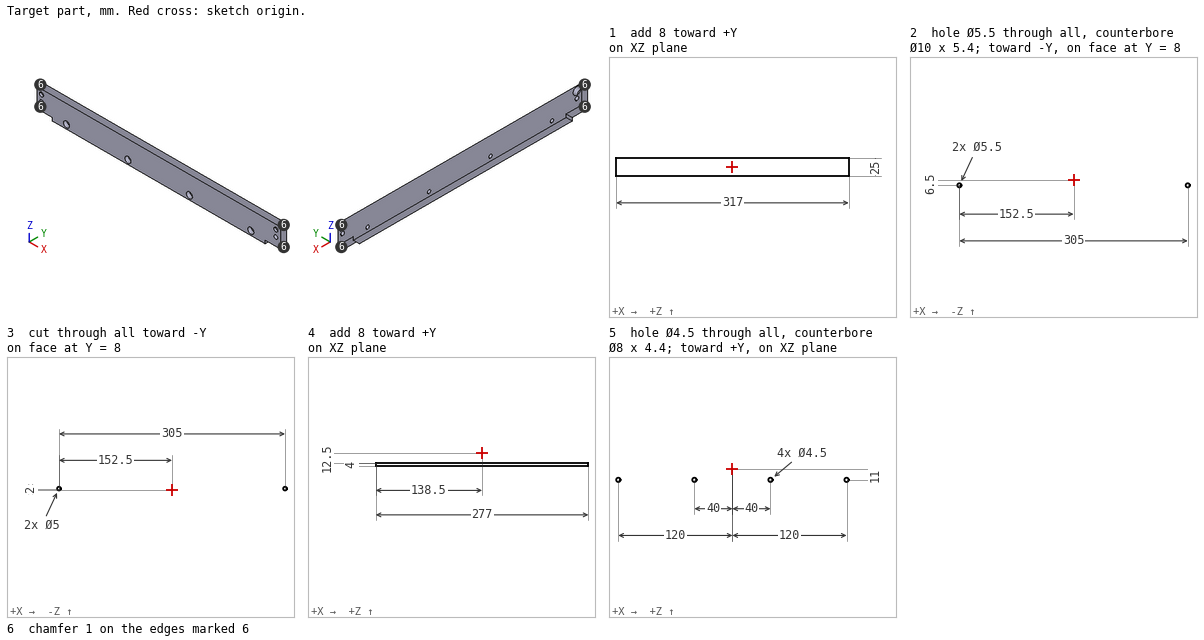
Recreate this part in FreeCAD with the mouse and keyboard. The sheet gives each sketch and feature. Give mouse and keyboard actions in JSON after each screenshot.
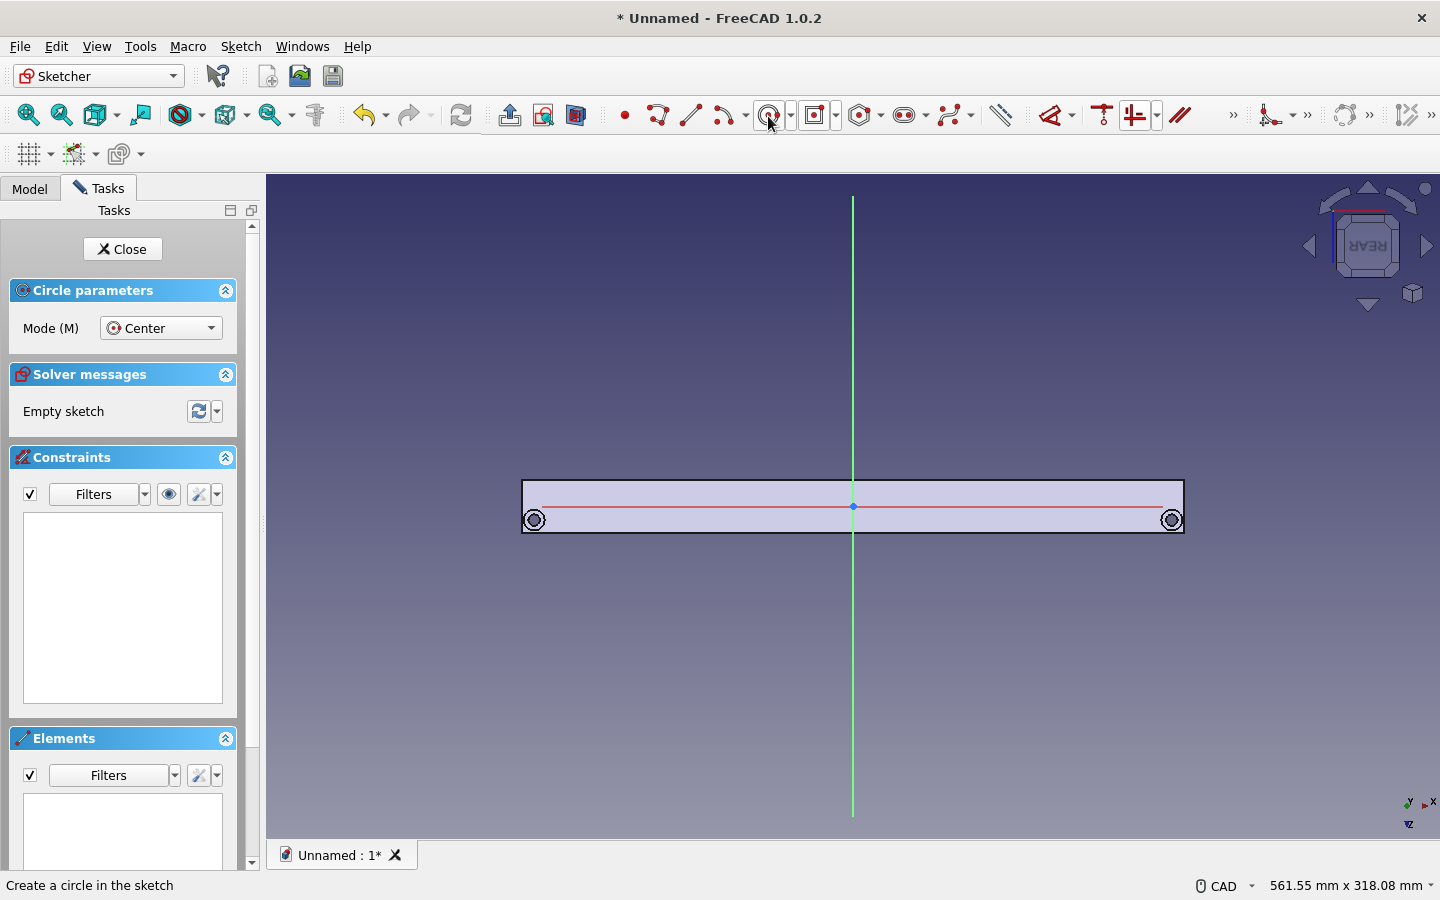
{"action": "scroll", "coordinate": [534, 502], "scroll_direction": "up", "scroll_amount": 8}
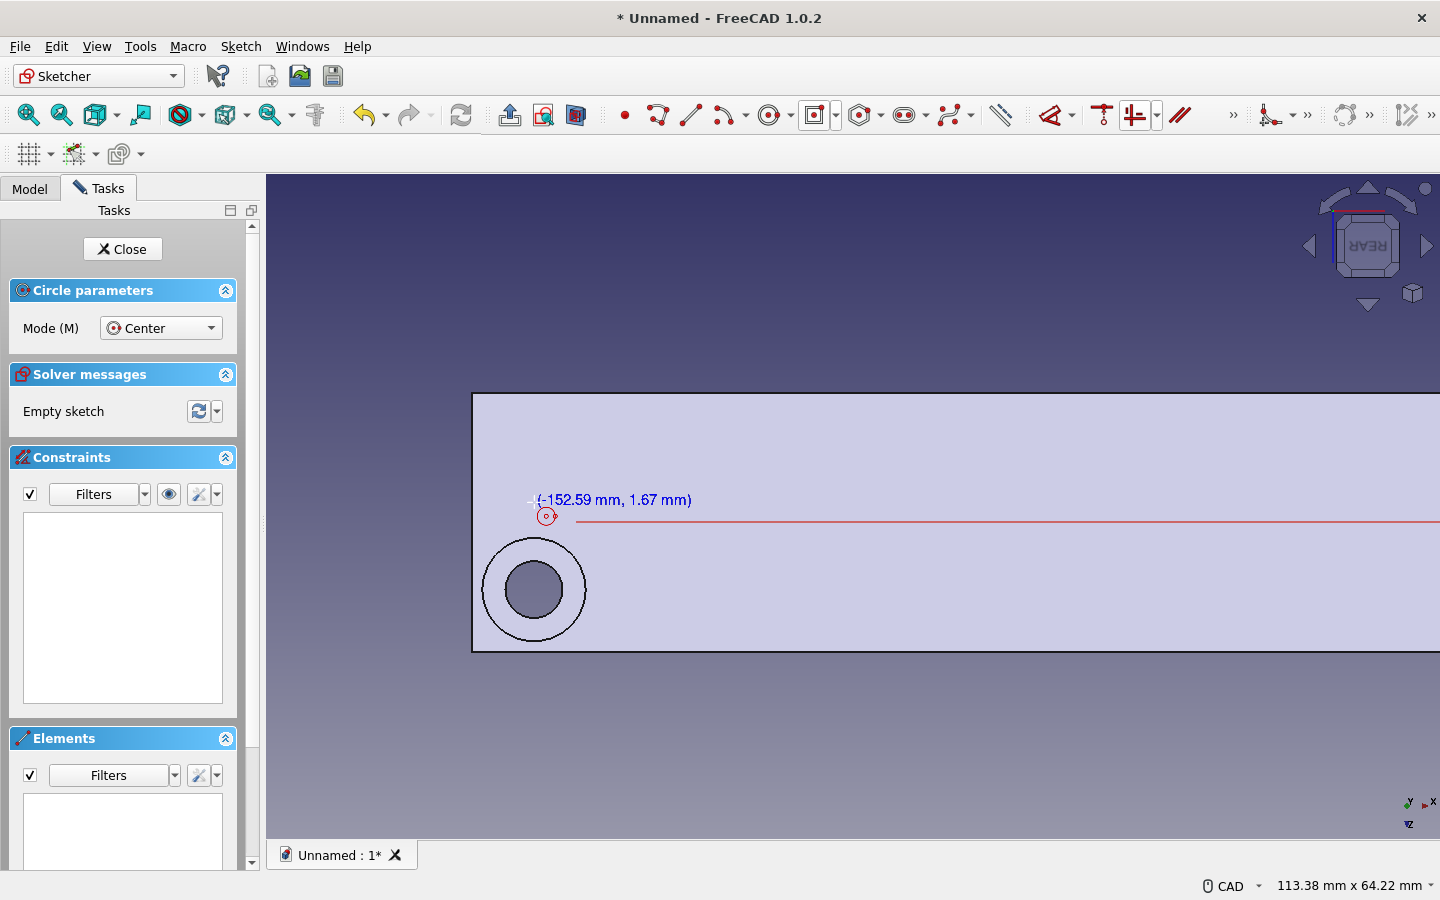
{"action": "left_click", "coordinate": [534, 502]}
{"action": "mouse_move", "coordinate": [552, 483]}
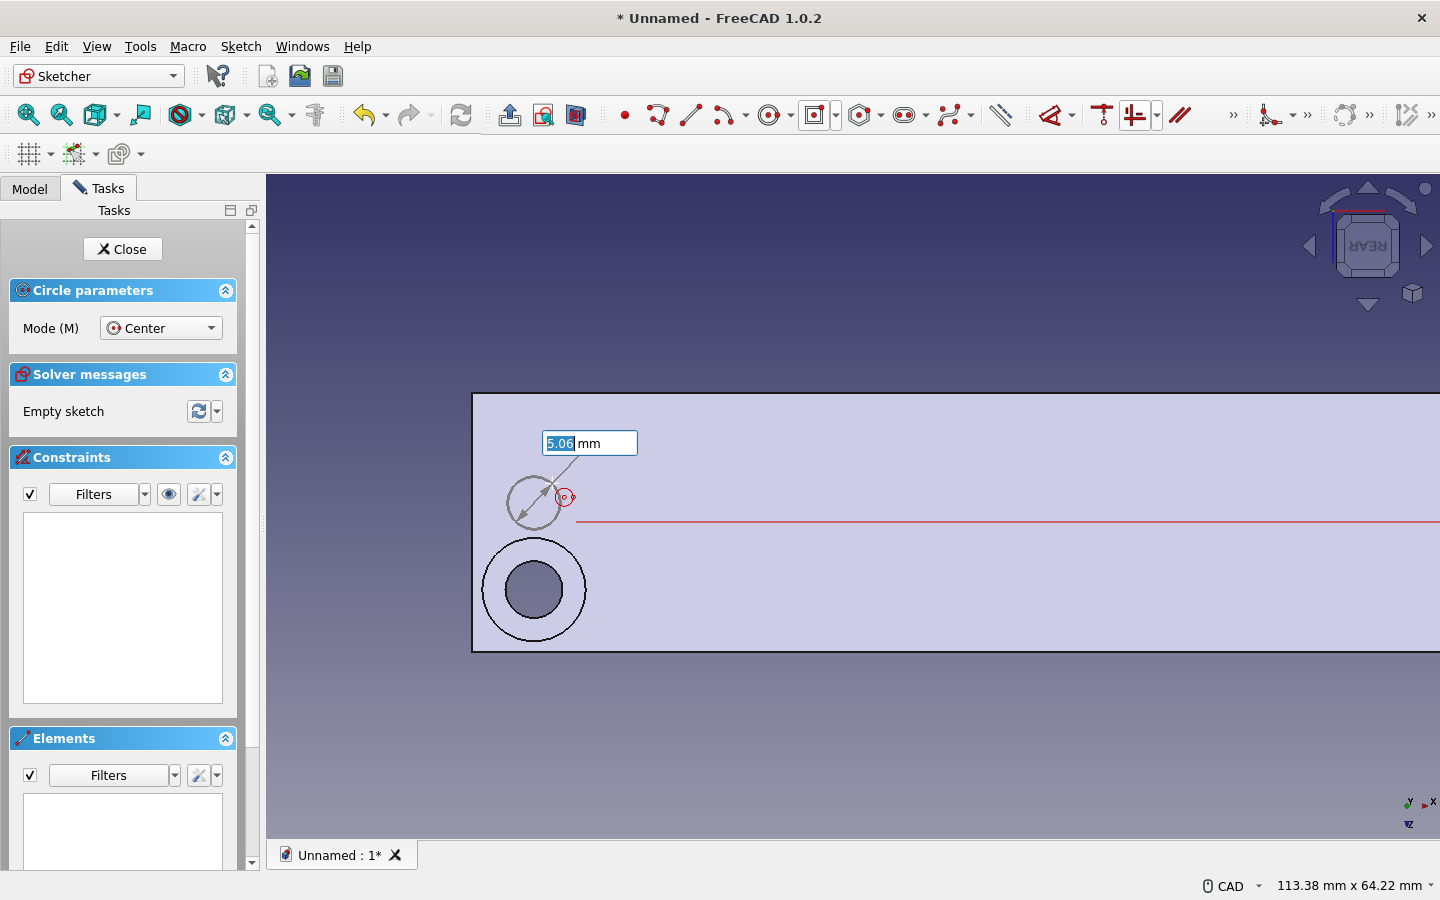
{"action": "type", "text": "5"}
{"action": "key", "text": "Return"}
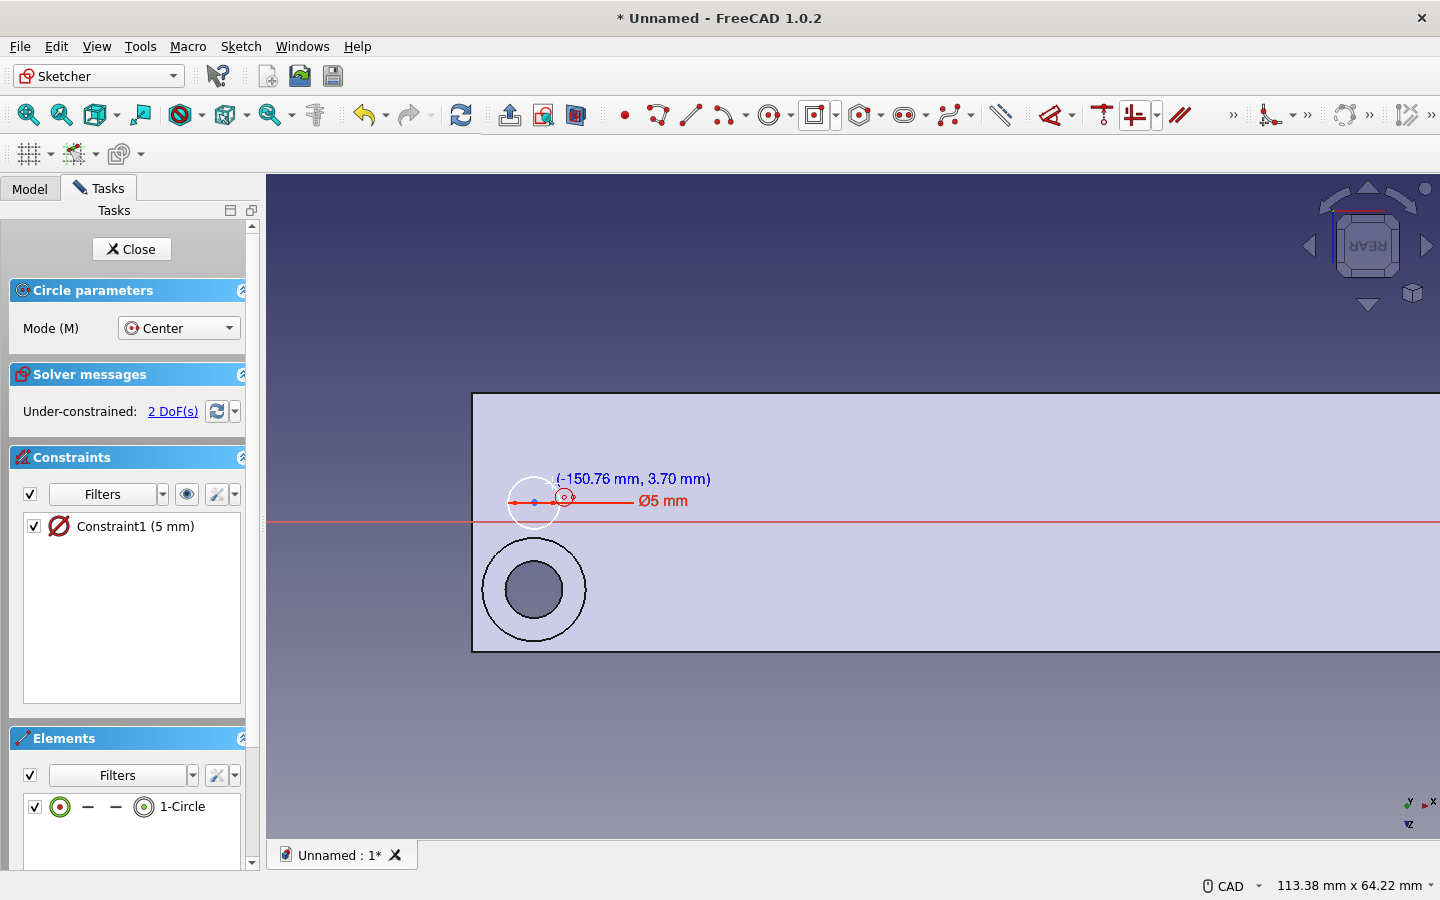
{"action": "scroll", "coordinate": [448, 508], "scroll_direction": "down", "scroll_amount": 8}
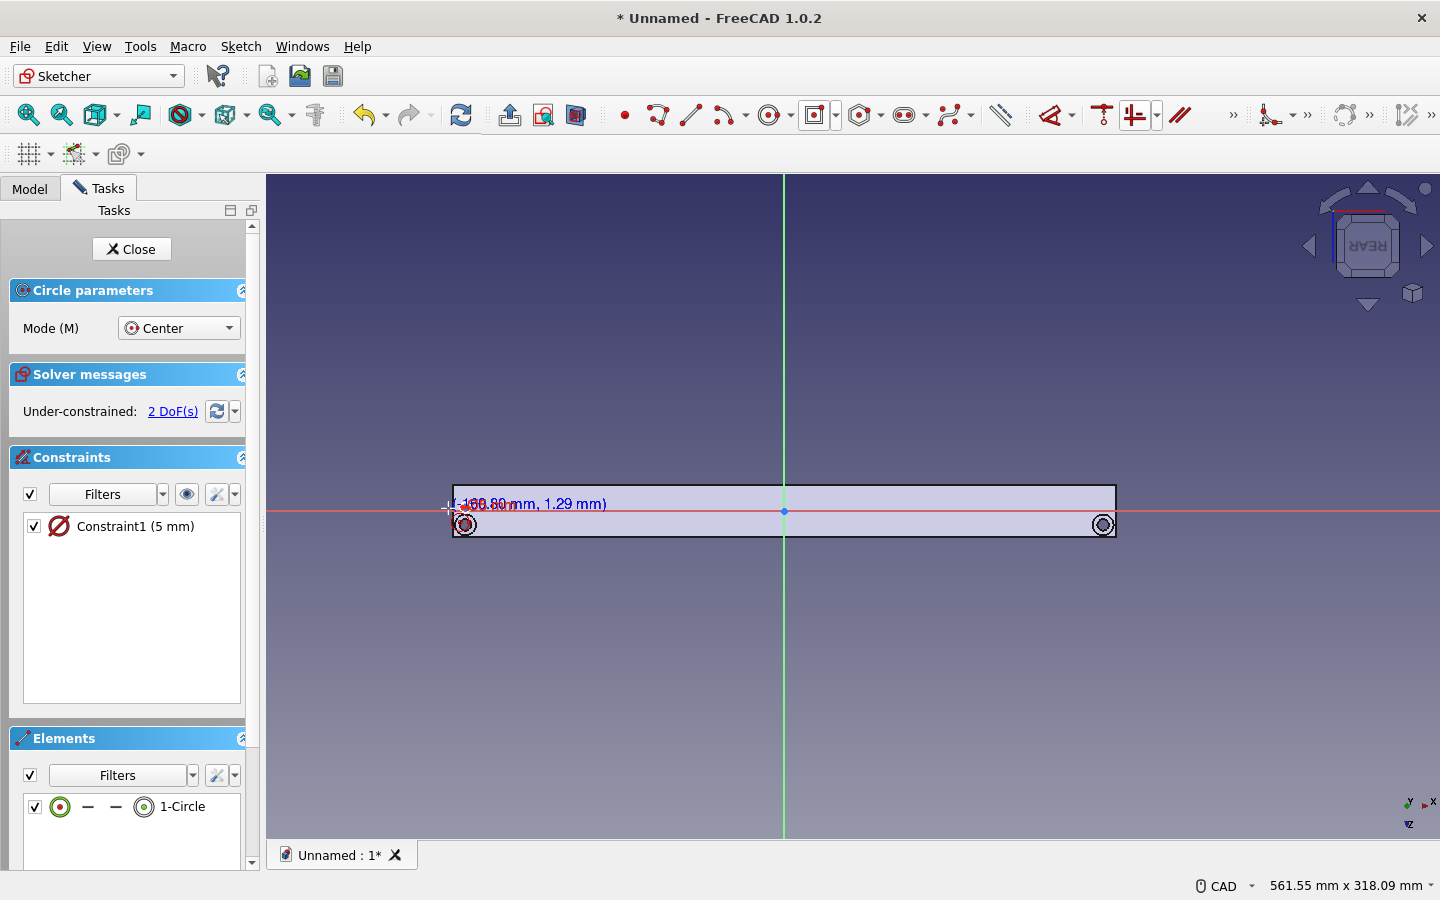
{"action": "scroll", "coordinate": [1103, 507], "scroll_direction": "up", "scroll_amount": 8}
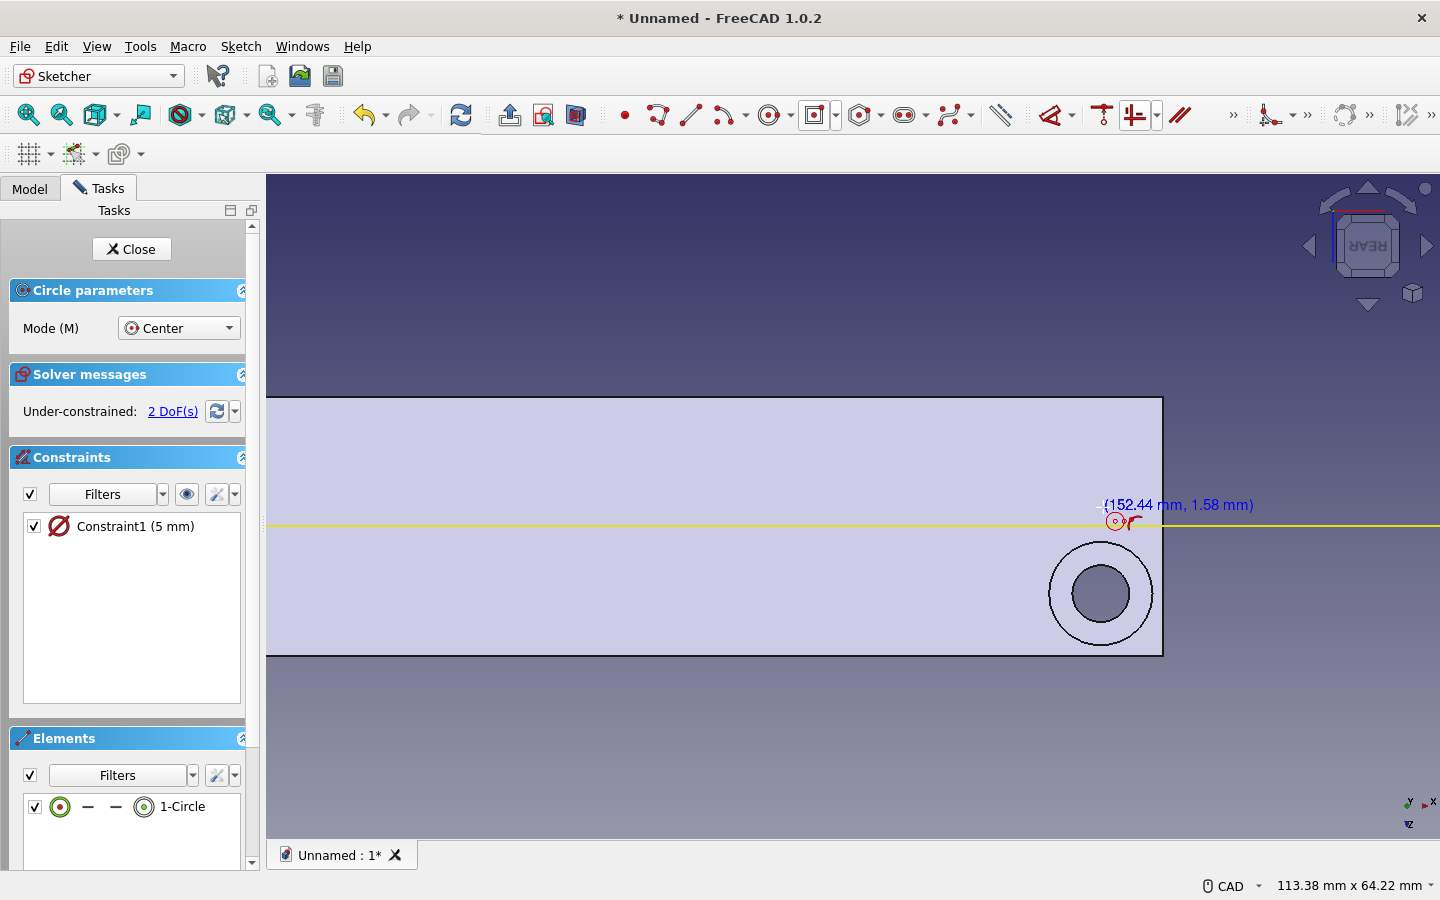
{"action": "left_click", "coordinate": [1101, 506]}
{"action": "mouse_move", "coordinate": [1119, 487]}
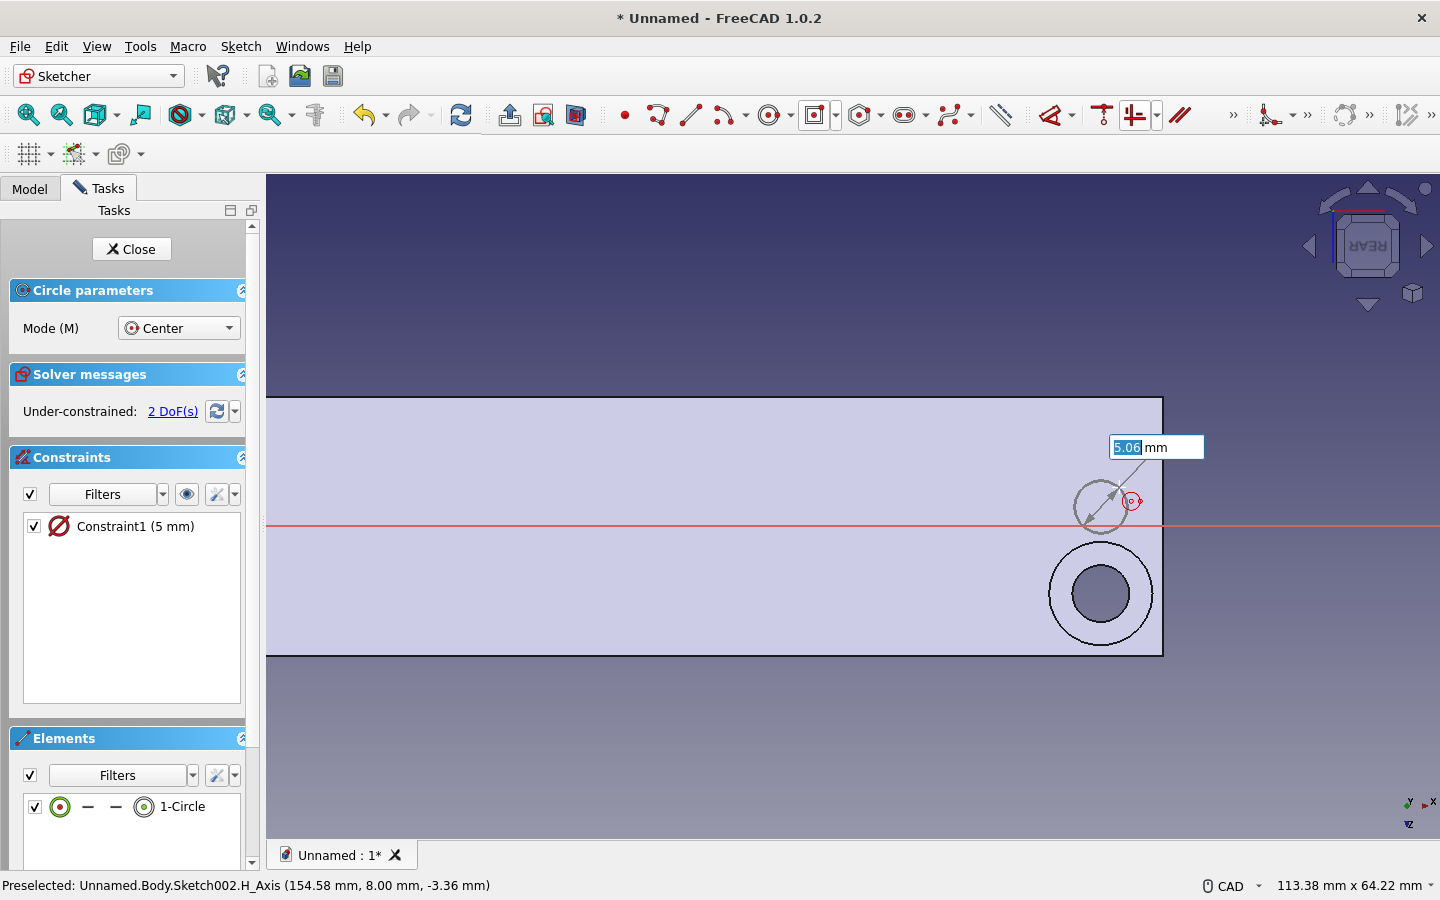
{"action": "type", "text": "5"}
{"action": "key", "text": "Return"}
{"action": "key", "text": "Escape"}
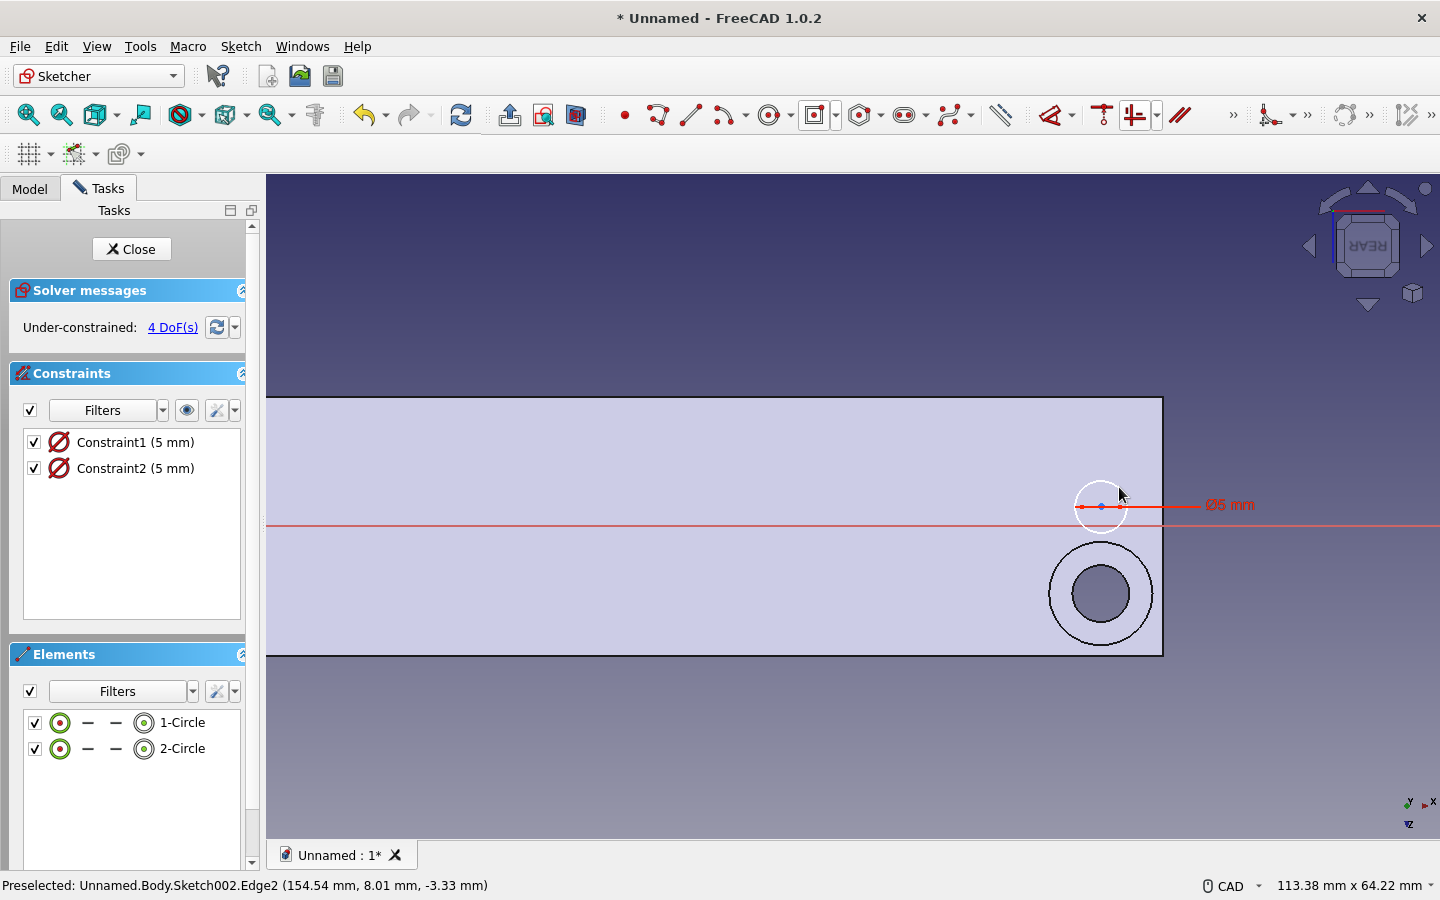
{"action": "scroll", "coordinate": [1104, 507], "scroll_direction": "down", "scroll_amount": 8}